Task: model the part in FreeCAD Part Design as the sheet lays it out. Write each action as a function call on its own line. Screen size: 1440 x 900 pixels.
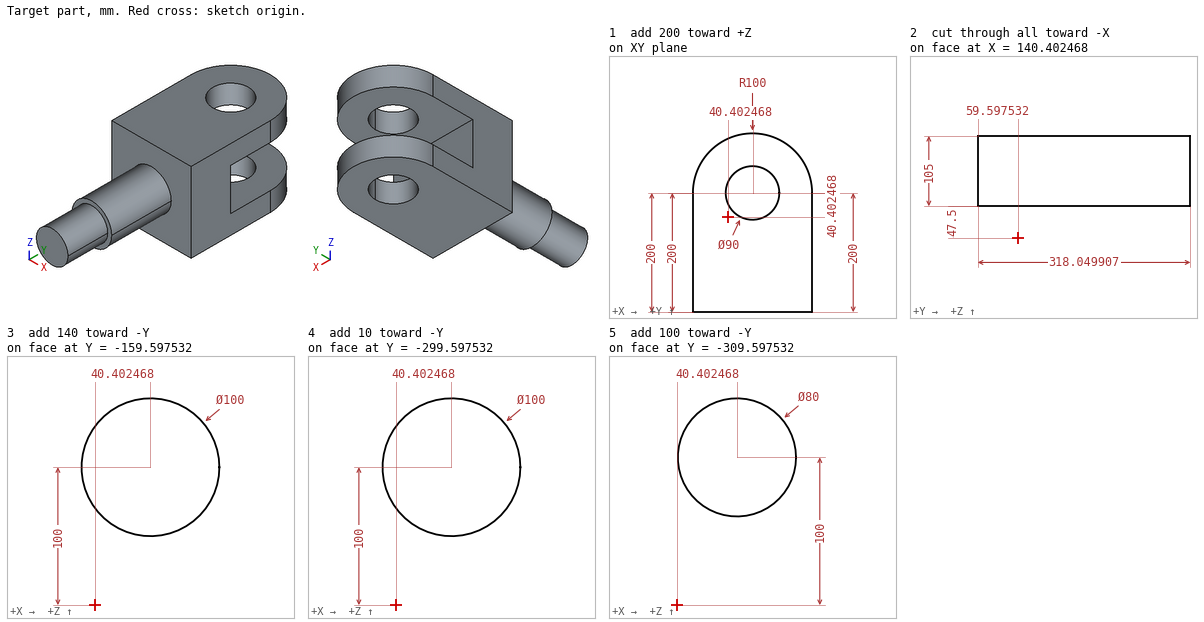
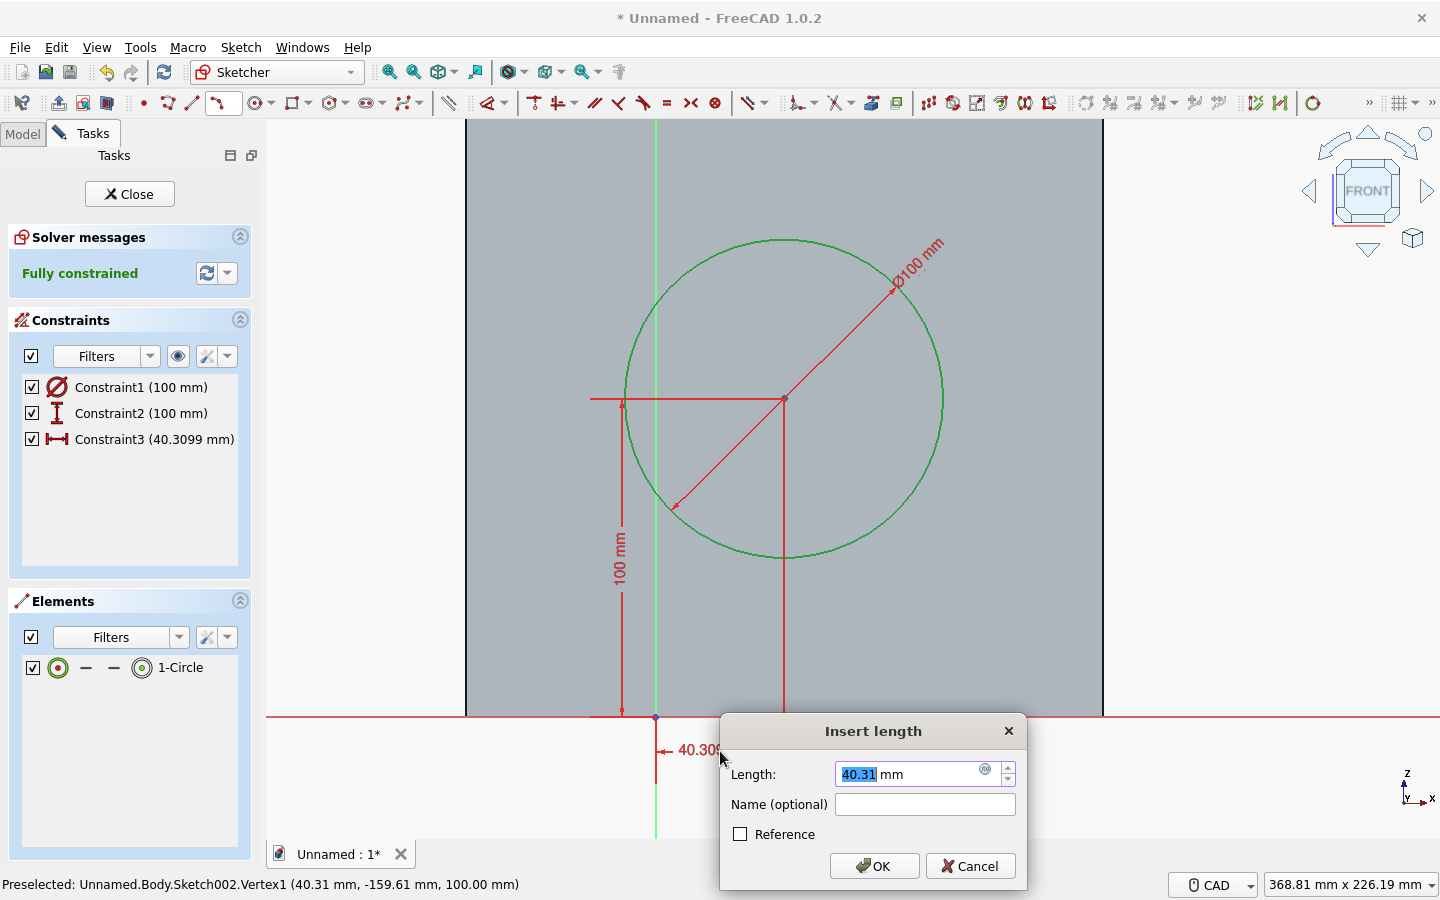
text(40.402468)
key(Return)
key(Escape)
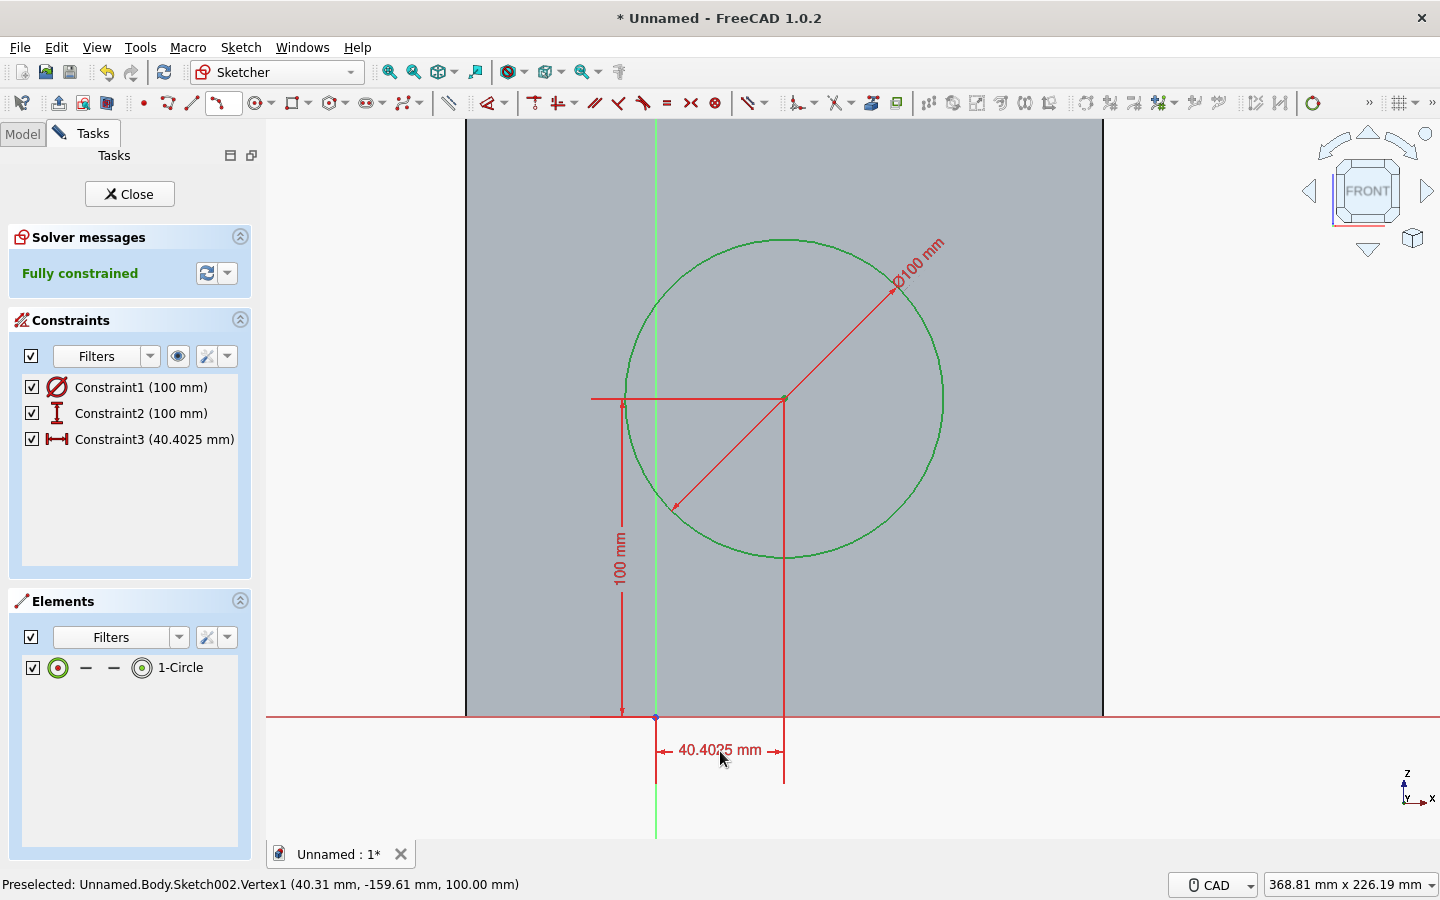
click(130, 194)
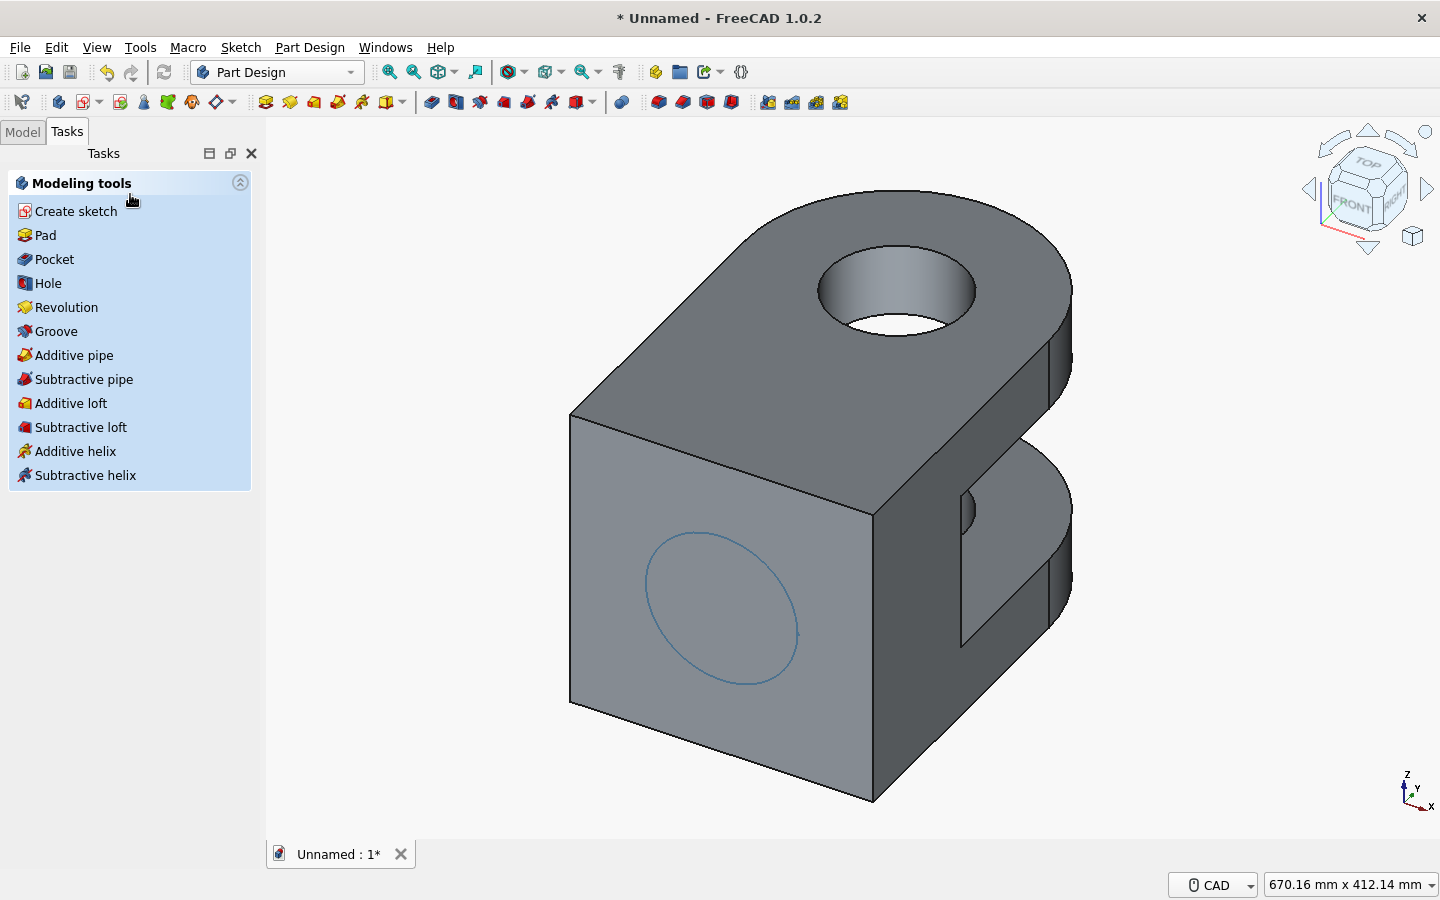
click(266, 102)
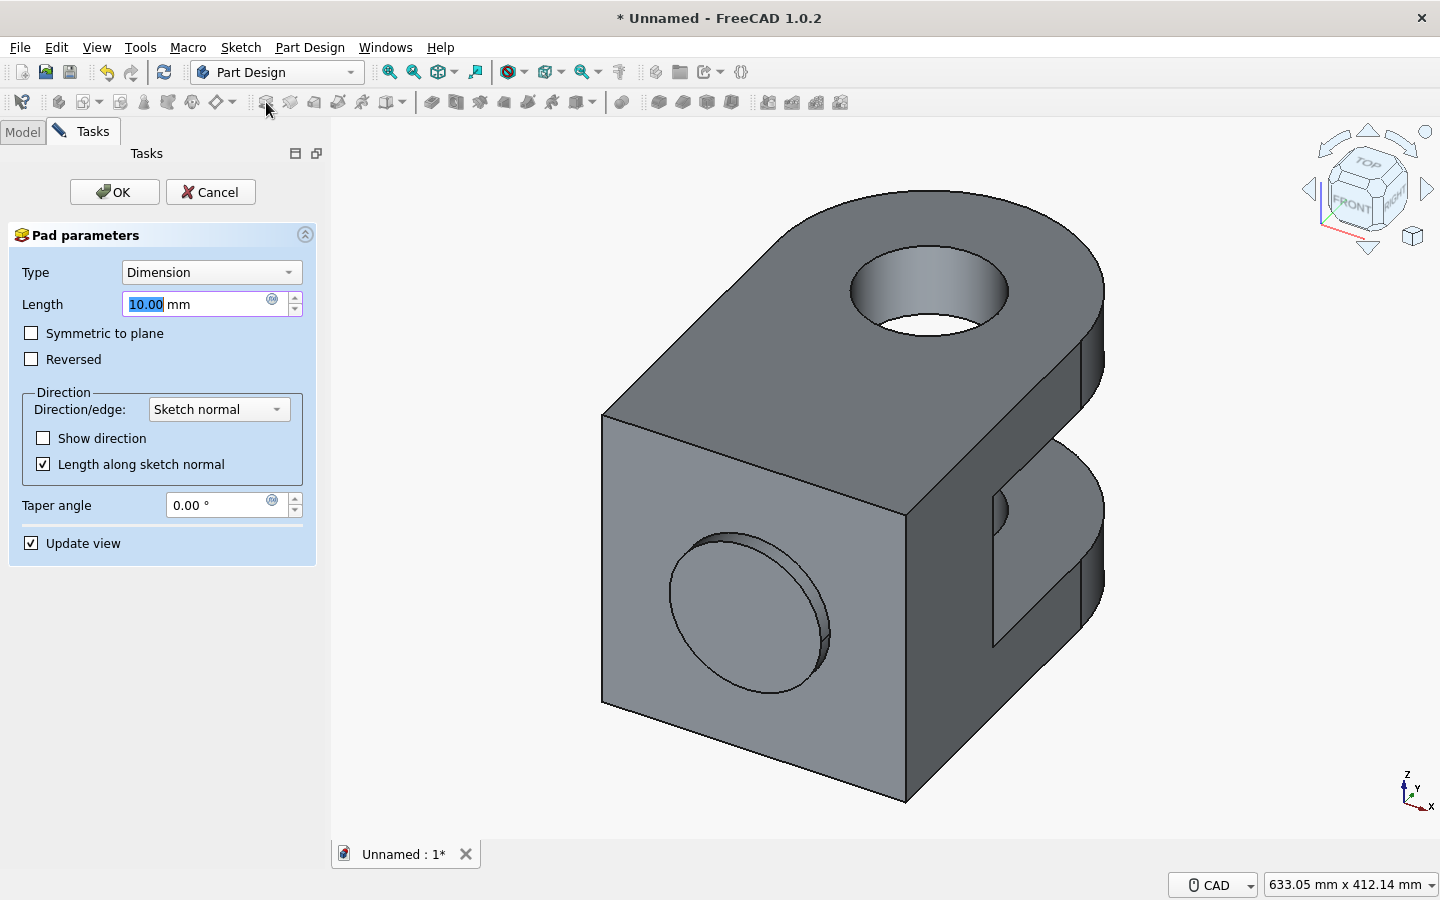
text(140)
key(Tab)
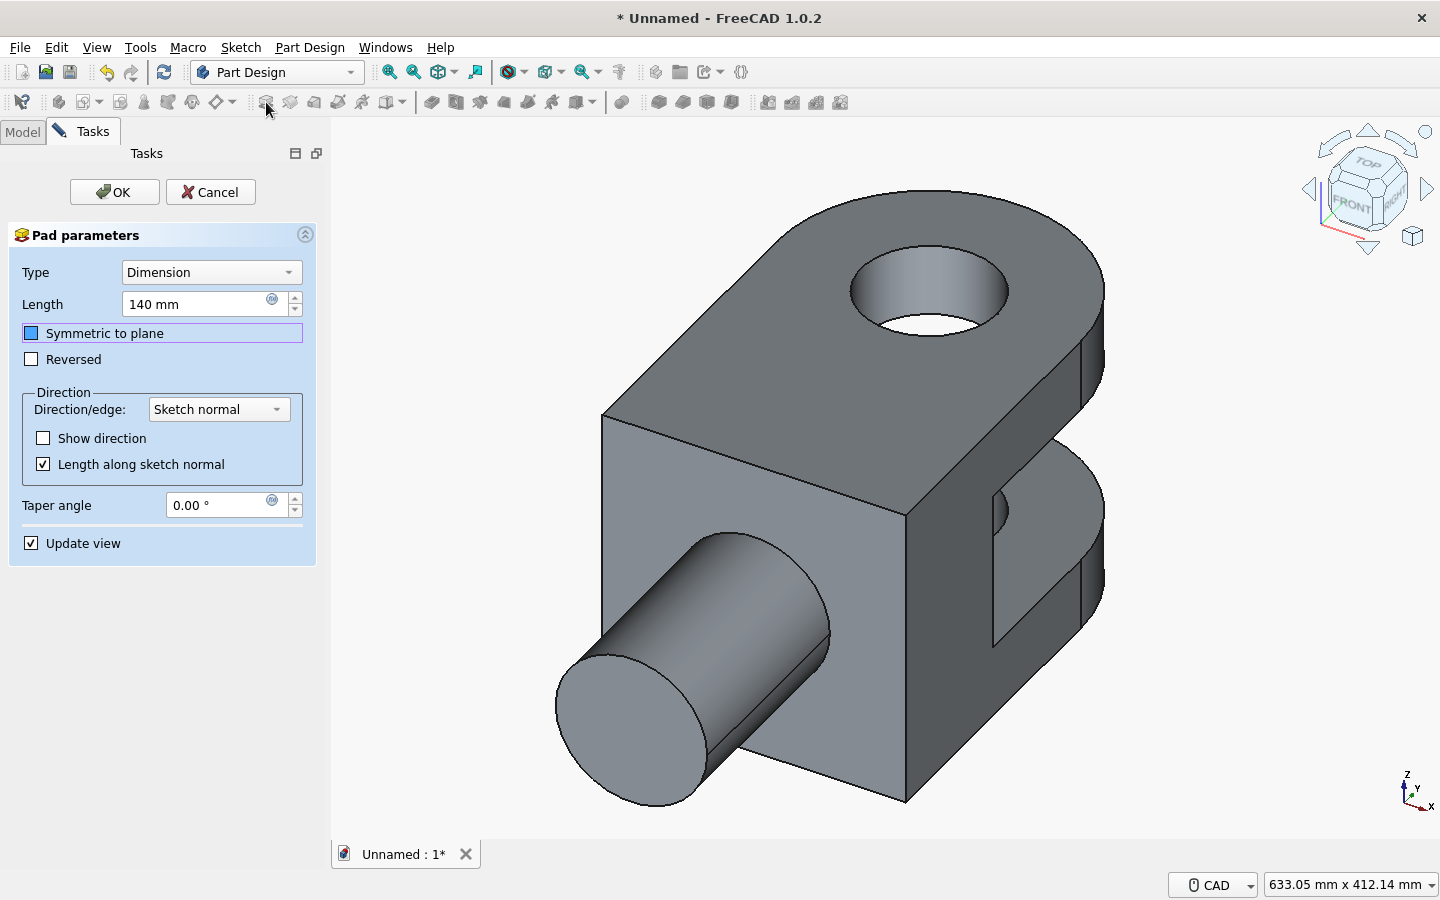
click(115, 192)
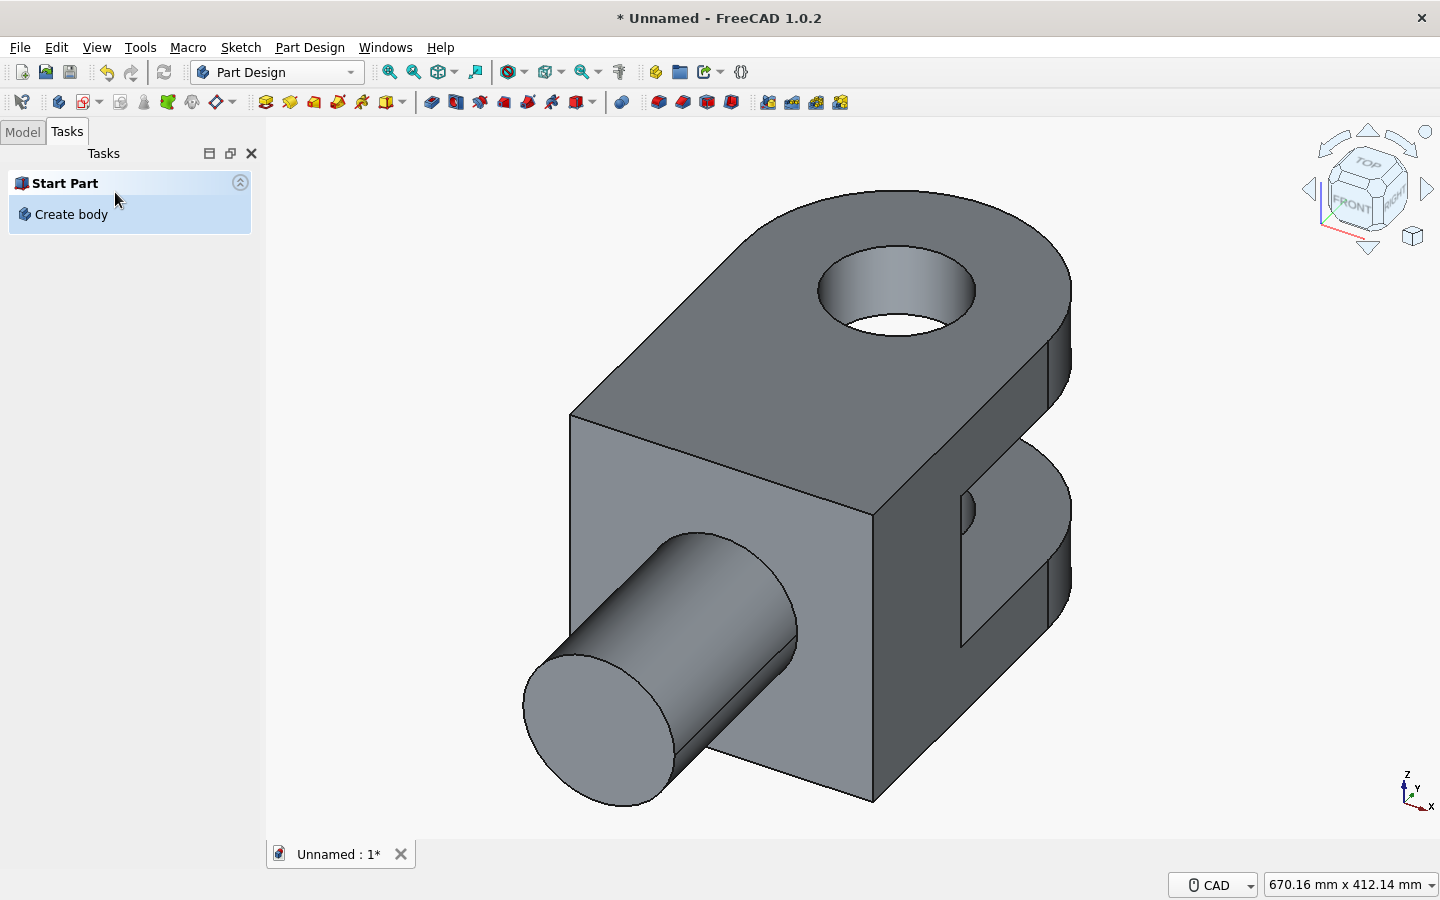
click(390, 72)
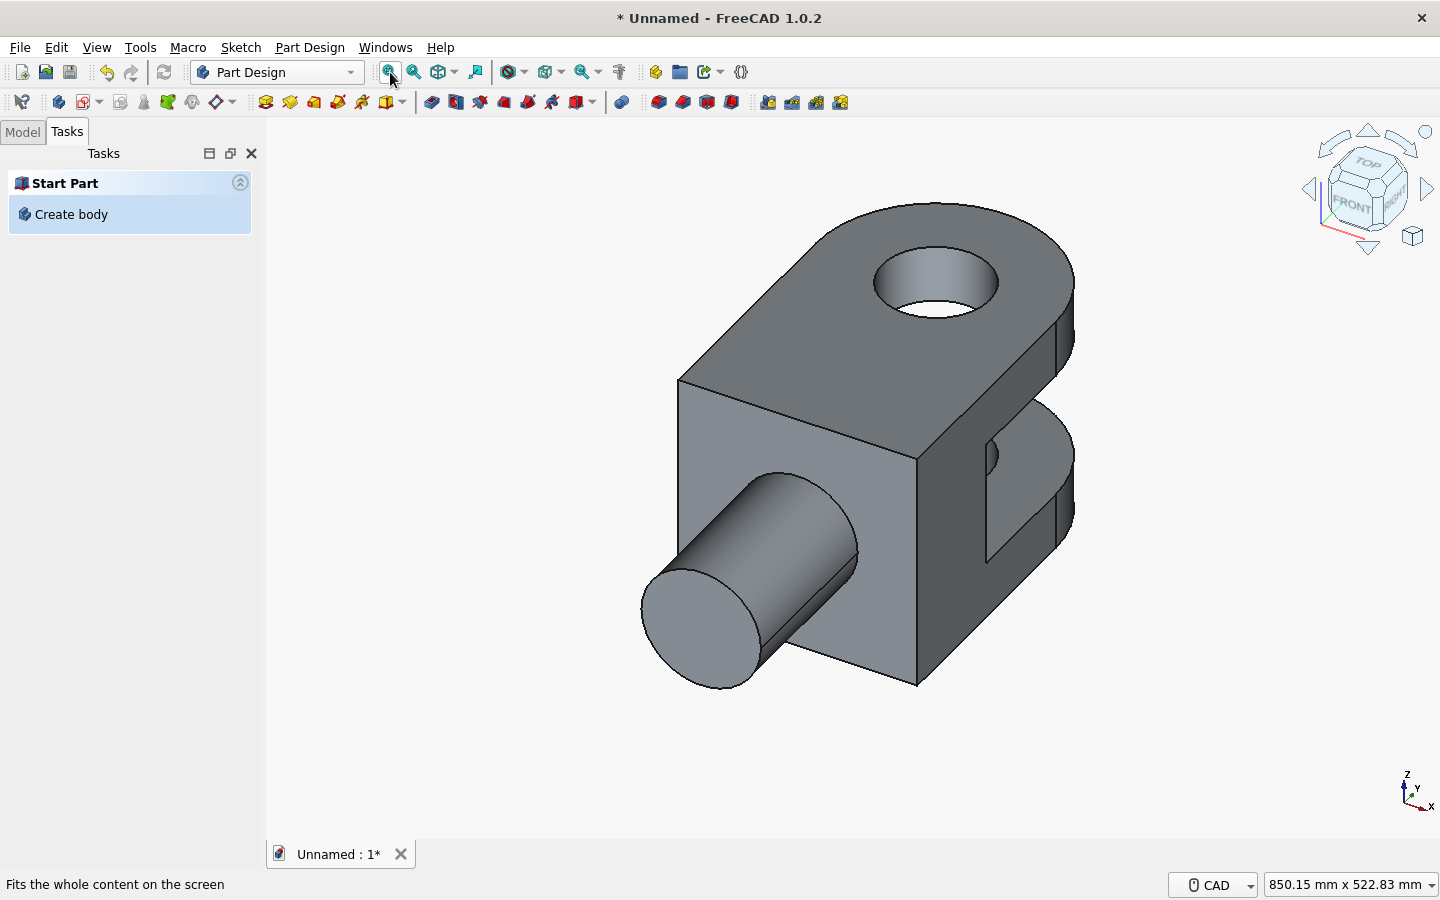
click(701, 628)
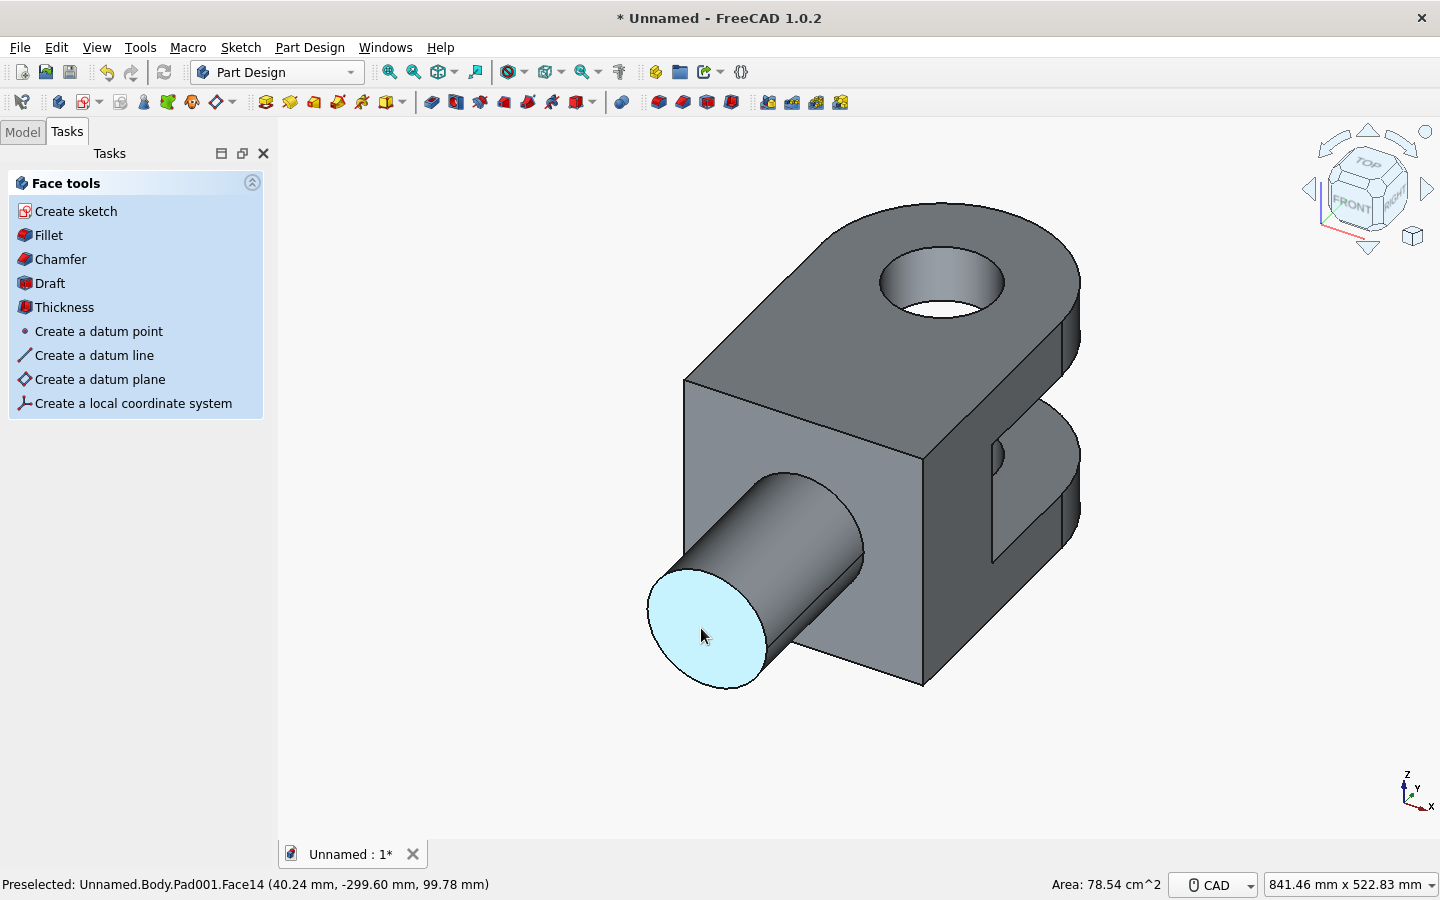
click(84, 102)